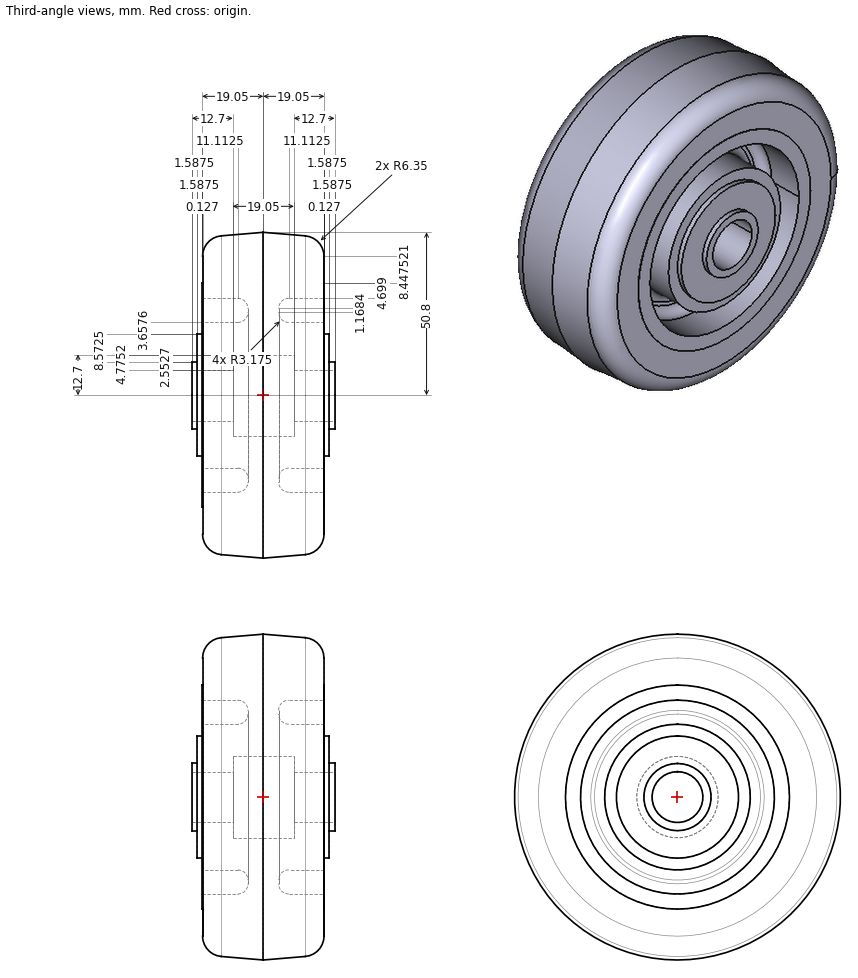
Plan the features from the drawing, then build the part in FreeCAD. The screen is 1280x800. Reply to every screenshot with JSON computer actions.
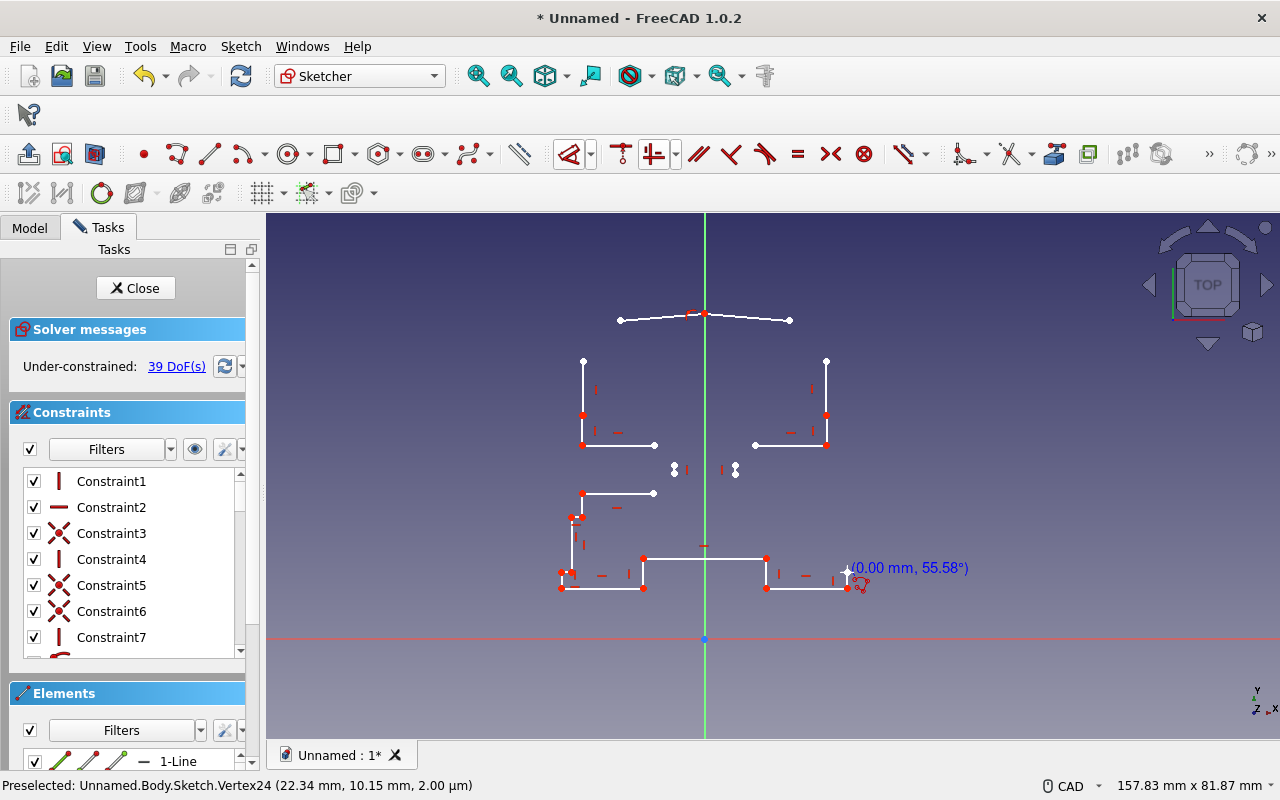
{"action": "scroll", "coordinate": [837, 572], "scroll_direction": "up", "scroll_amount": 3}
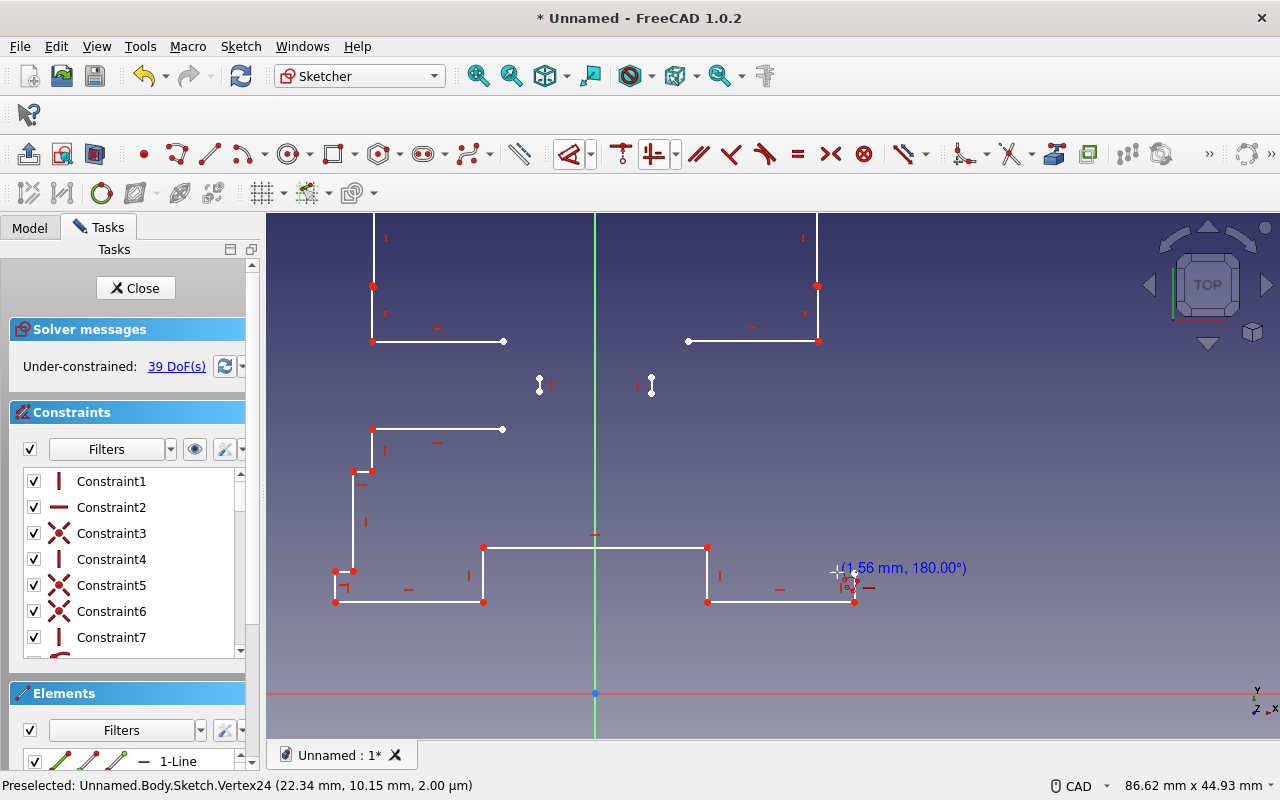
{"action": "left_click", "coordinate": [837, 571]}
{"action": "left_click", "coordinate": [837, 471]}
{"action": "left_click", "coordinate": [818, 471]}
{"action": "left_click", "coordinate": [818, 428]}
{"action": "left_click", "coordinate": [688, 428]}
{"action": "right_click", "coordinate": [688, 428]}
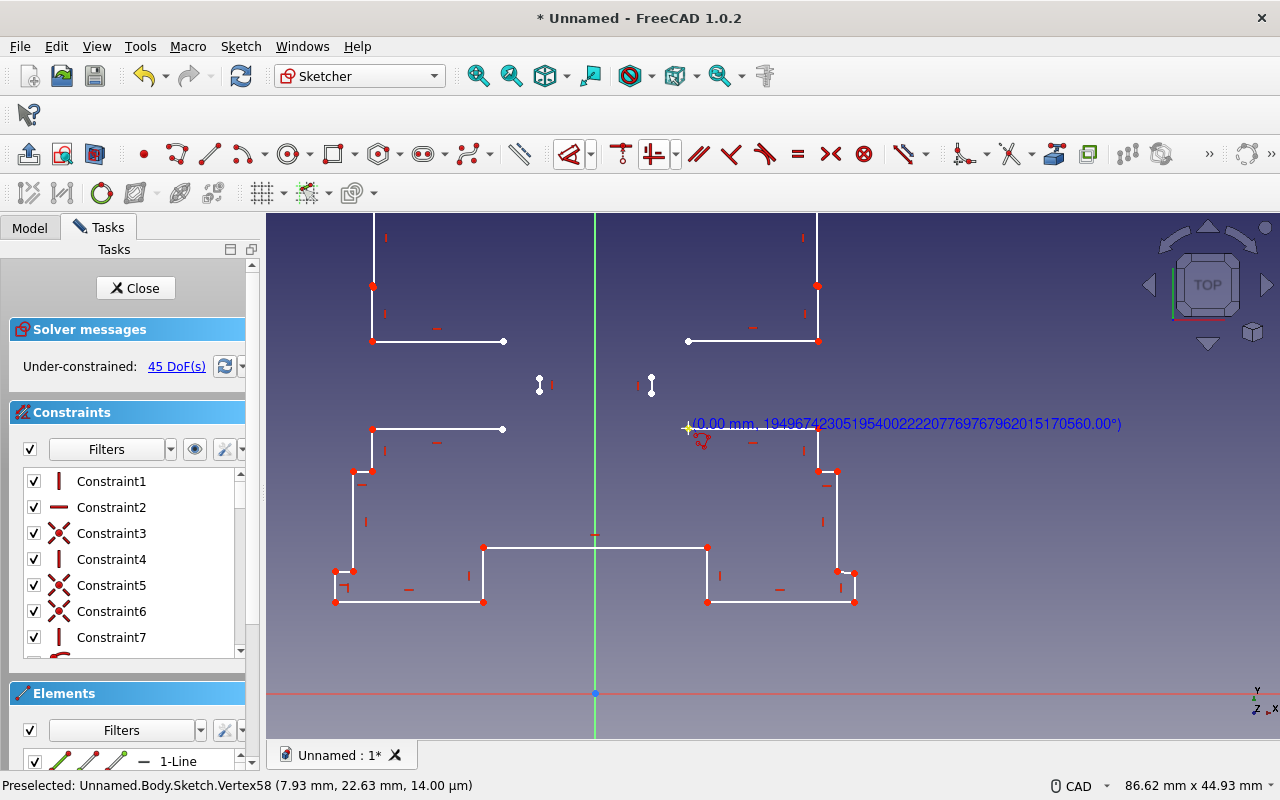
{"action": "key", "text": "g 3 a"}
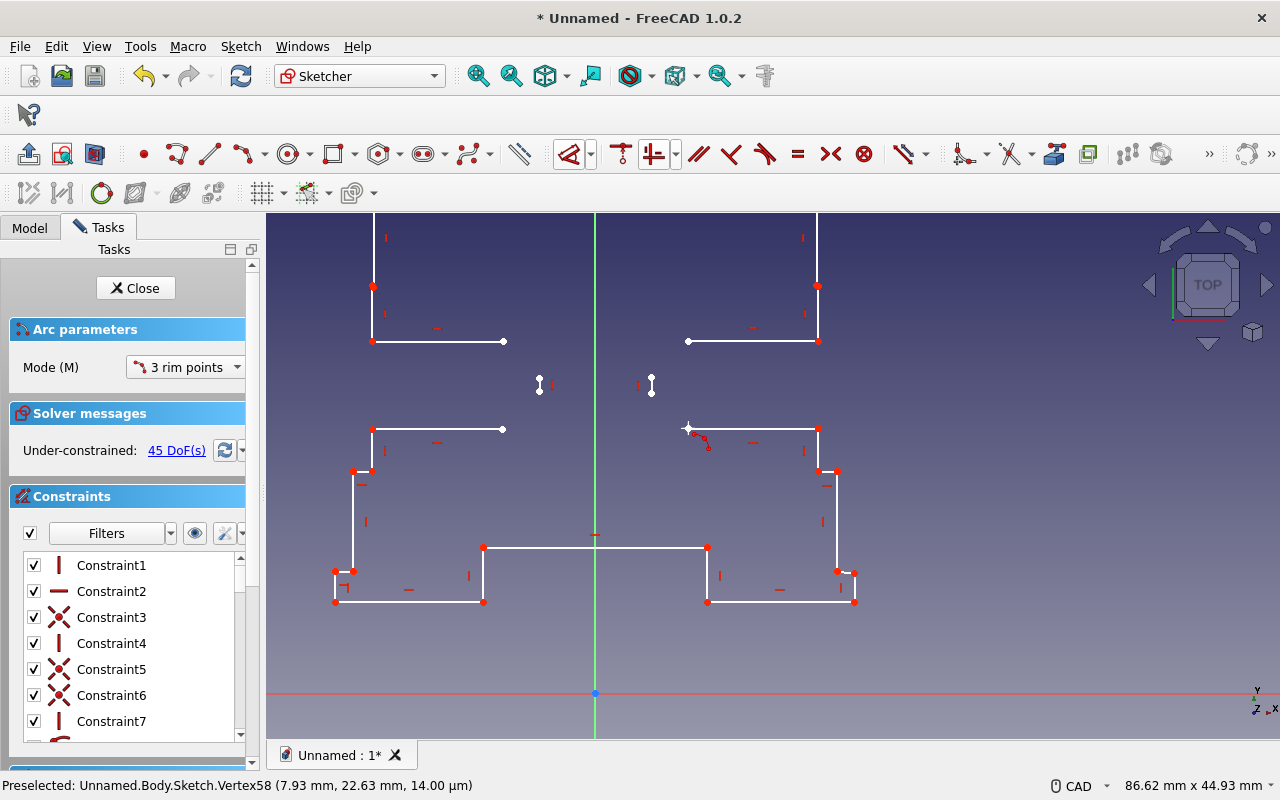
{"action": "scroll", "coordinate": [651, 377], "scroll_direction": "up", "scroll_amount": 5}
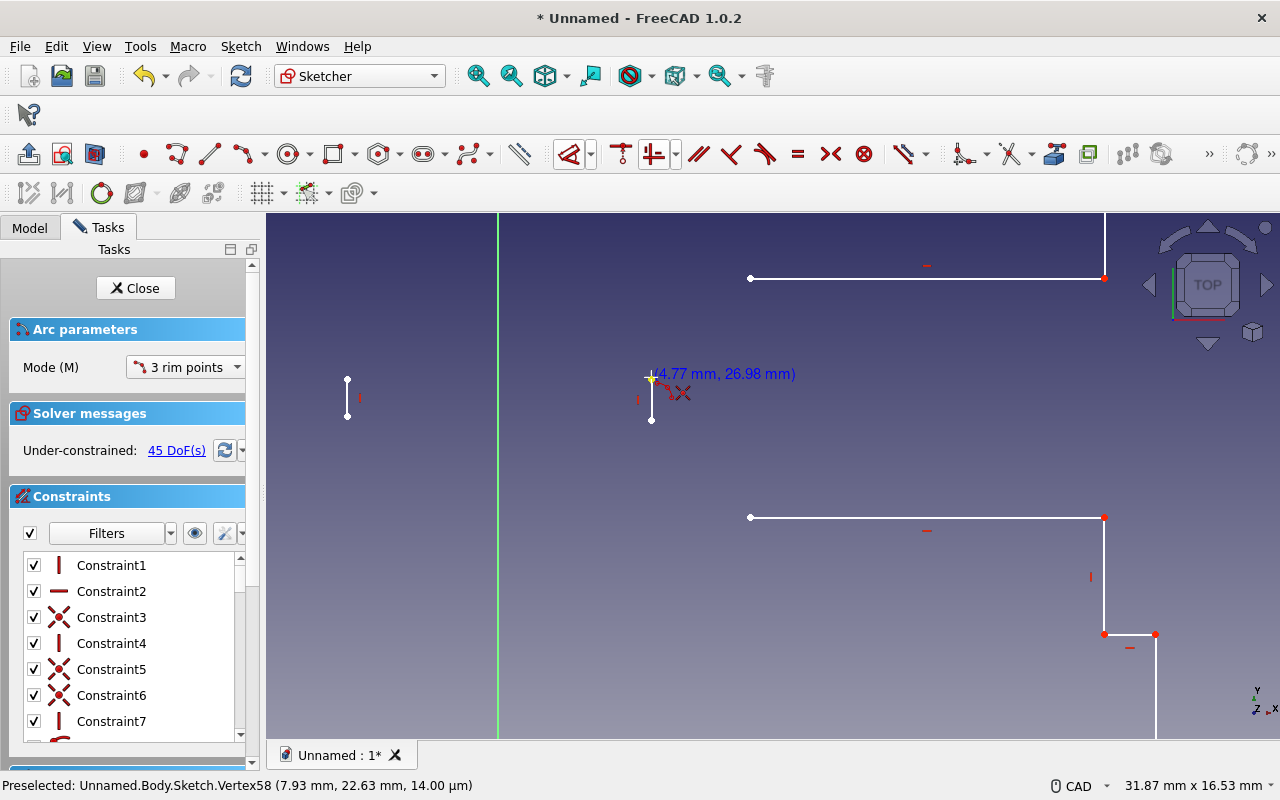
{"action": "left_click", "coordinate": [652, 379]}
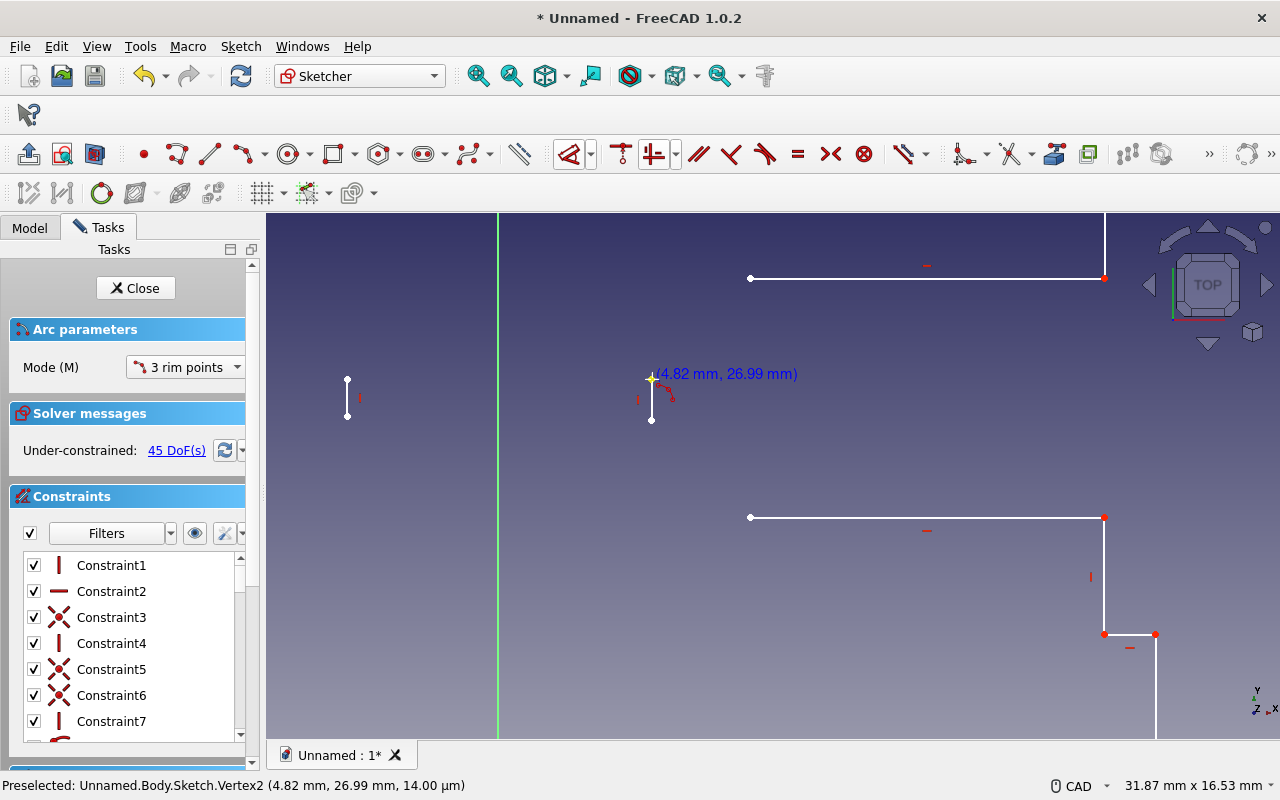
{"action": "scroll", "coordinate": [757, 488], "scroll_direction": "down", "scroll_amount": 8}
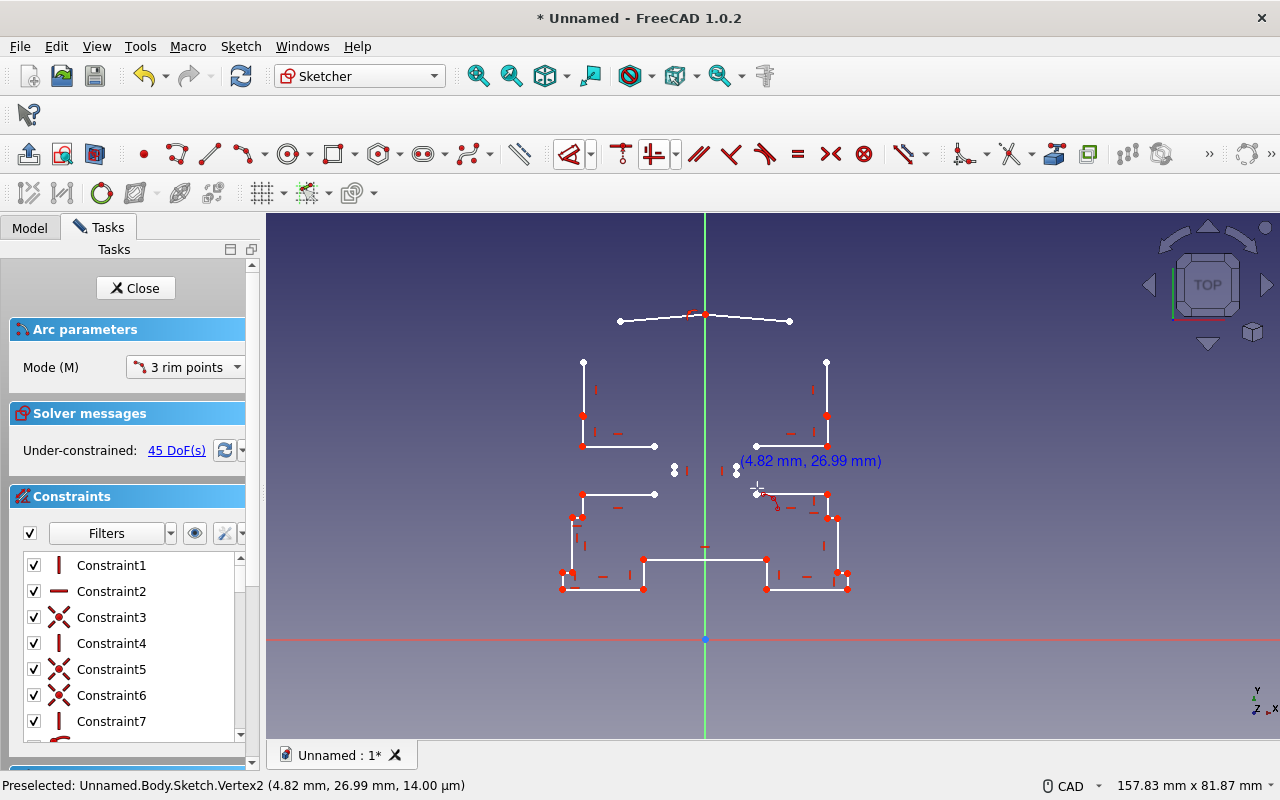
{"action": "left_click", "coordinate": [756, 446]}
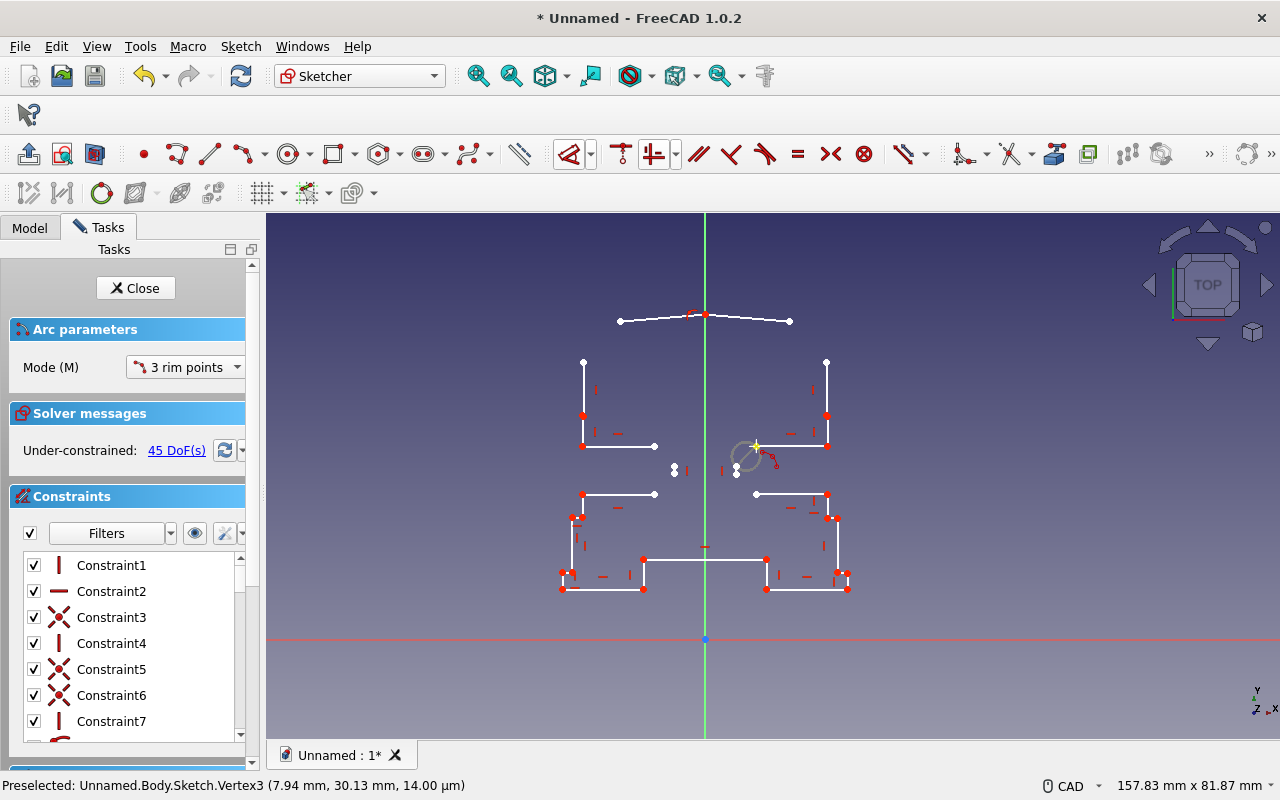
{"action": "scroll", "coordinate": [742, 452], "scroll_direction": "up", "scroll_amount": 5}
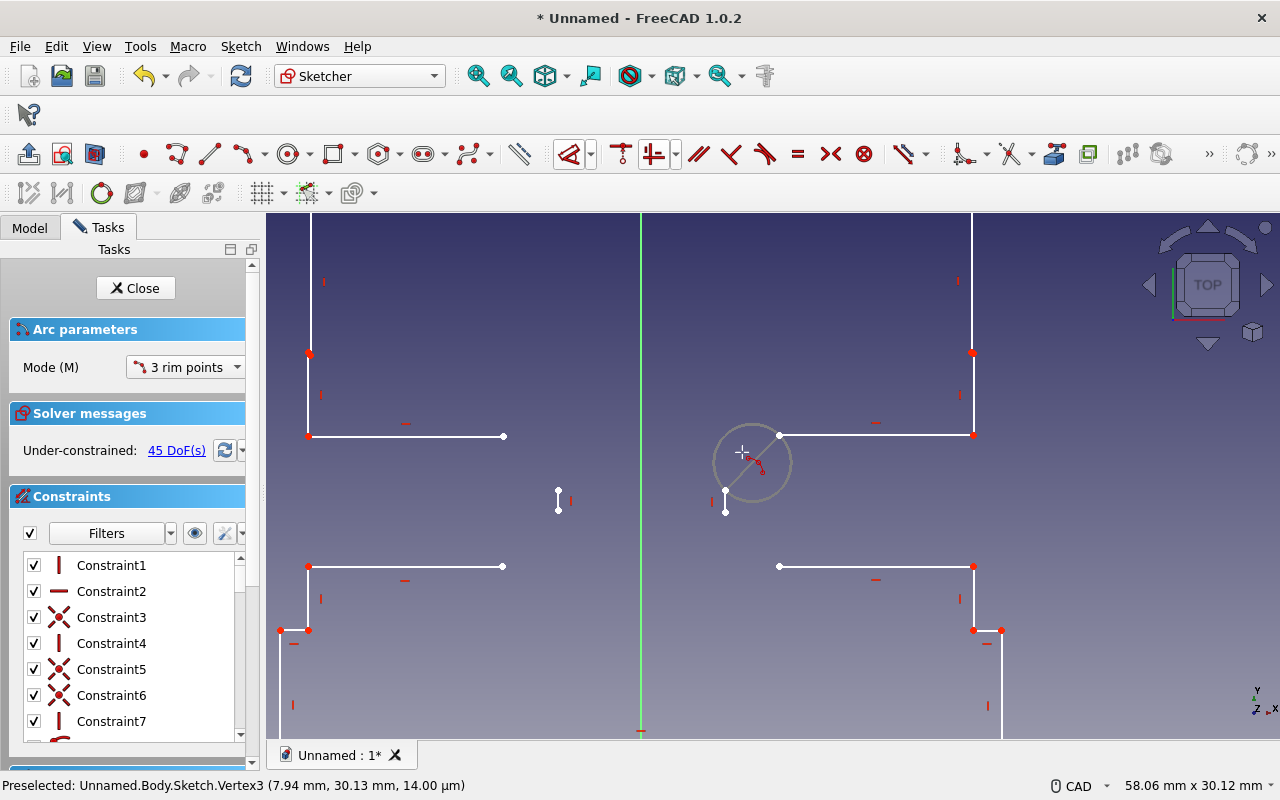
{"action": "left_click", "coordinate": [741, 450]}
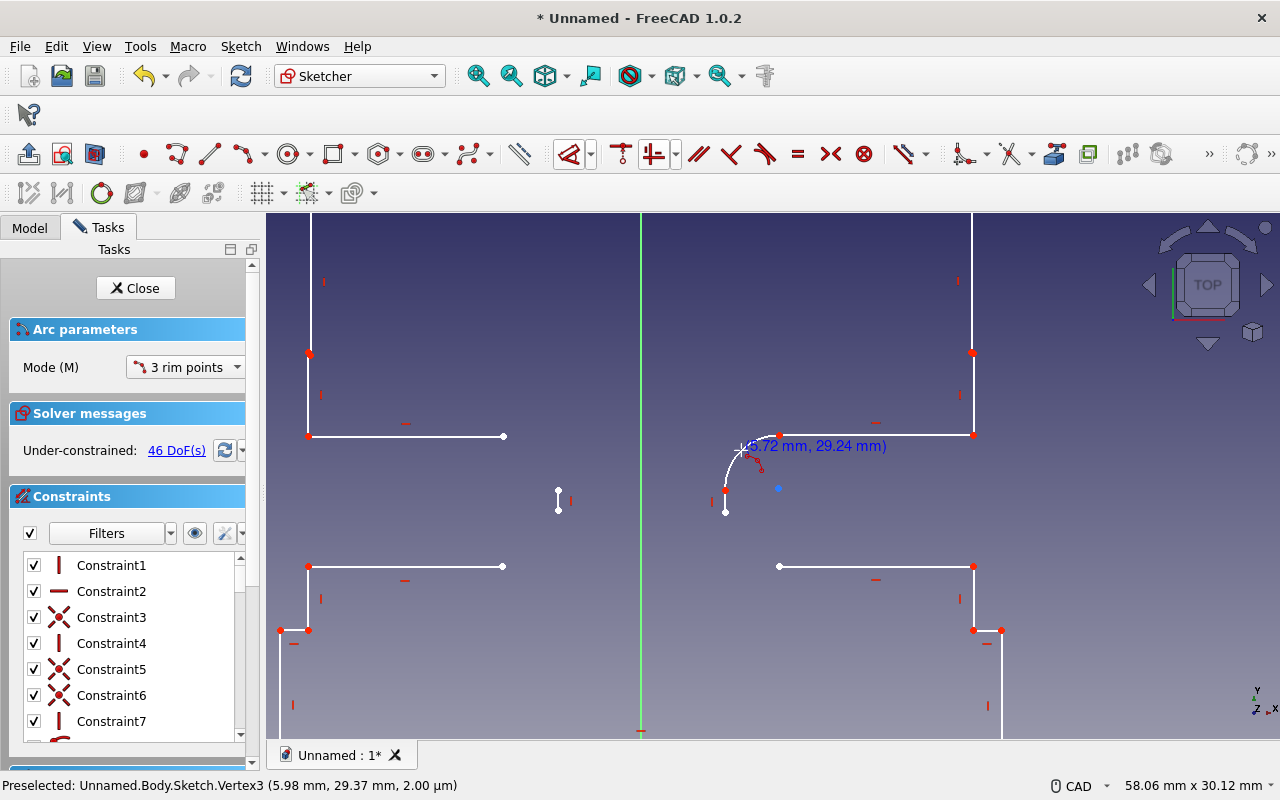
{"action": "scroll", "coordinate": [741, 451], "scroll_direction": "down", "scroll_amount": 5}